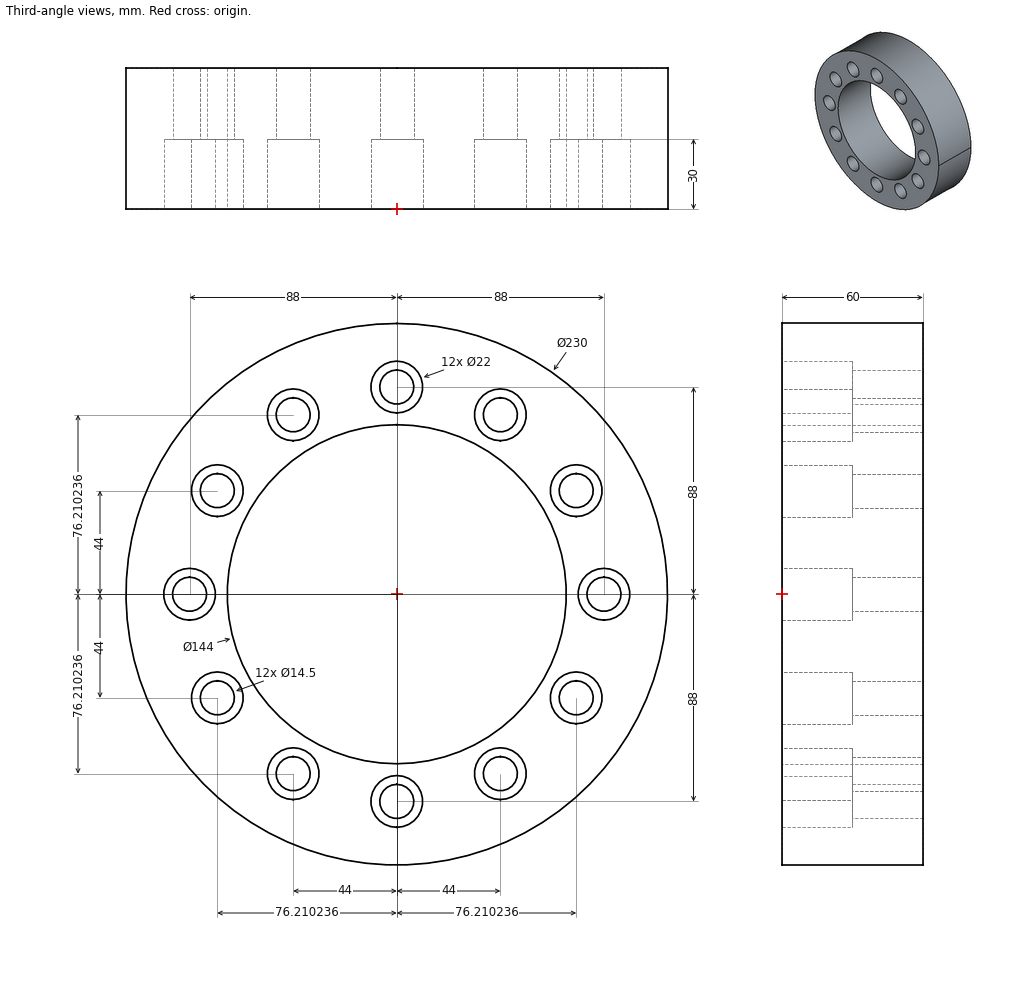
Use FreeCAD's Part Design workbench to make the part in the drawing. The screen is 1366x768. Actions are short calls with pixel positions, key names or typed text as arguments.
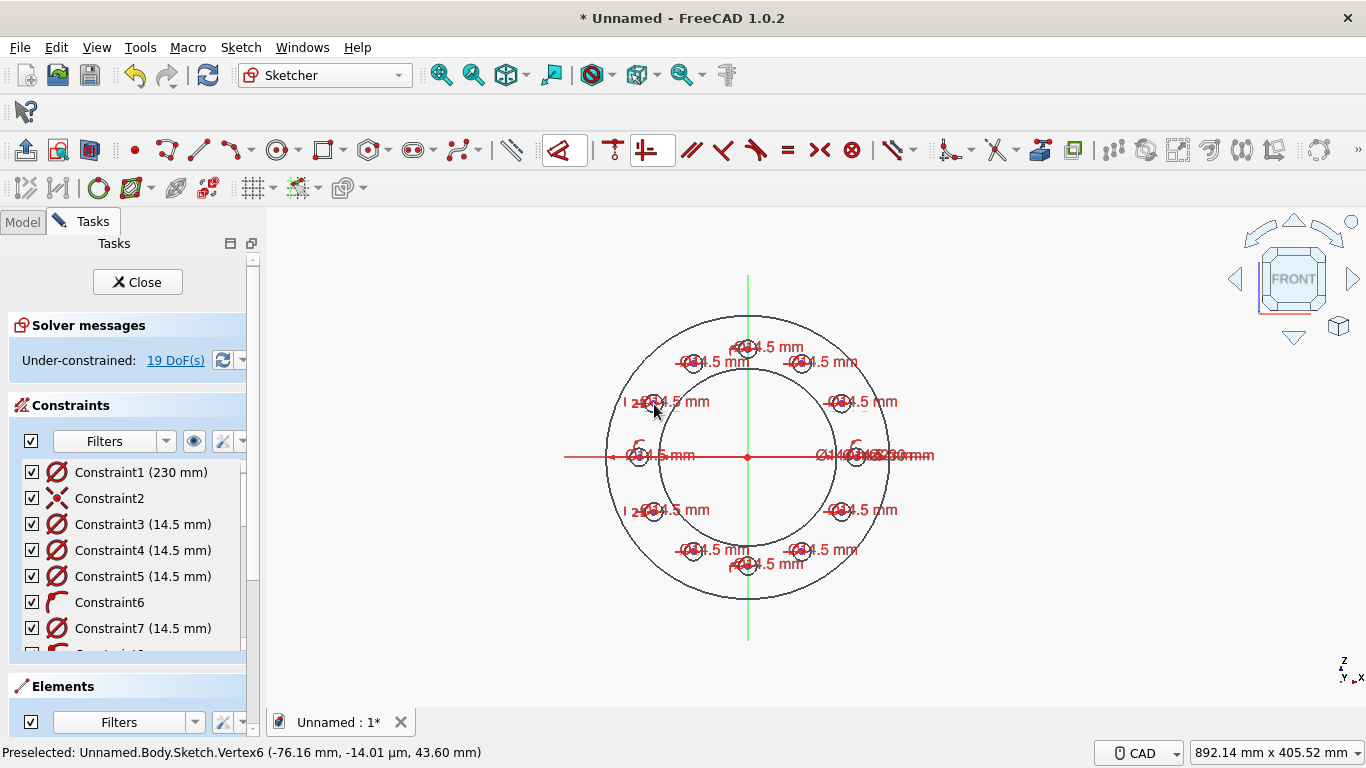
click(694, 552)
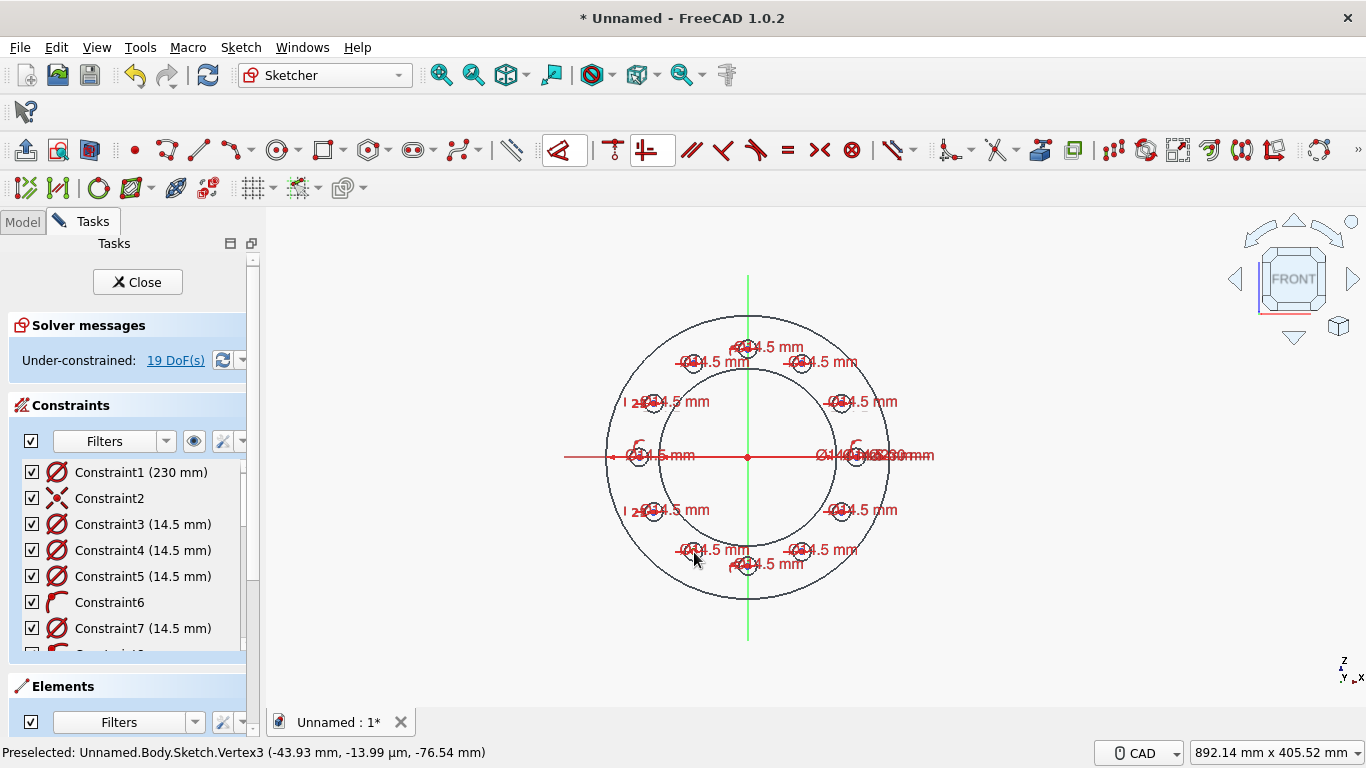
click(694, 364)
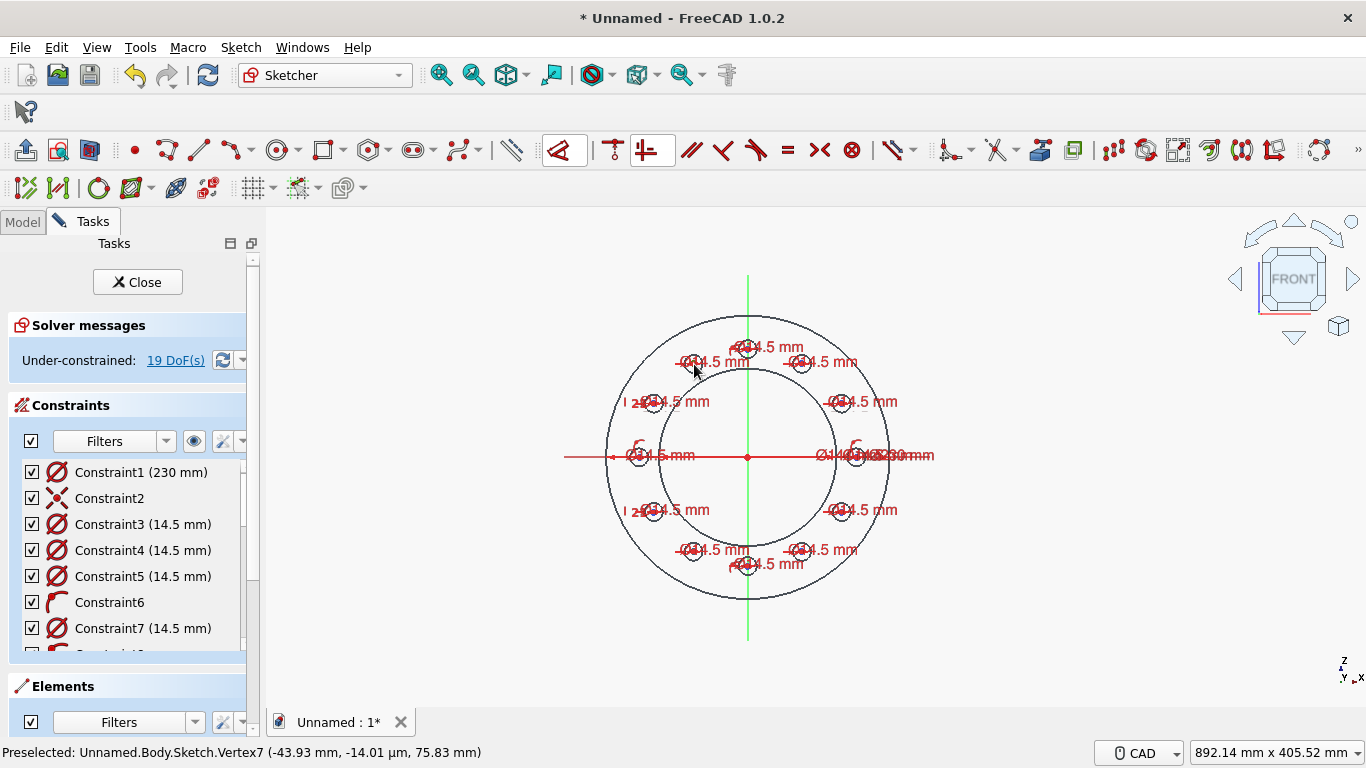
key(v)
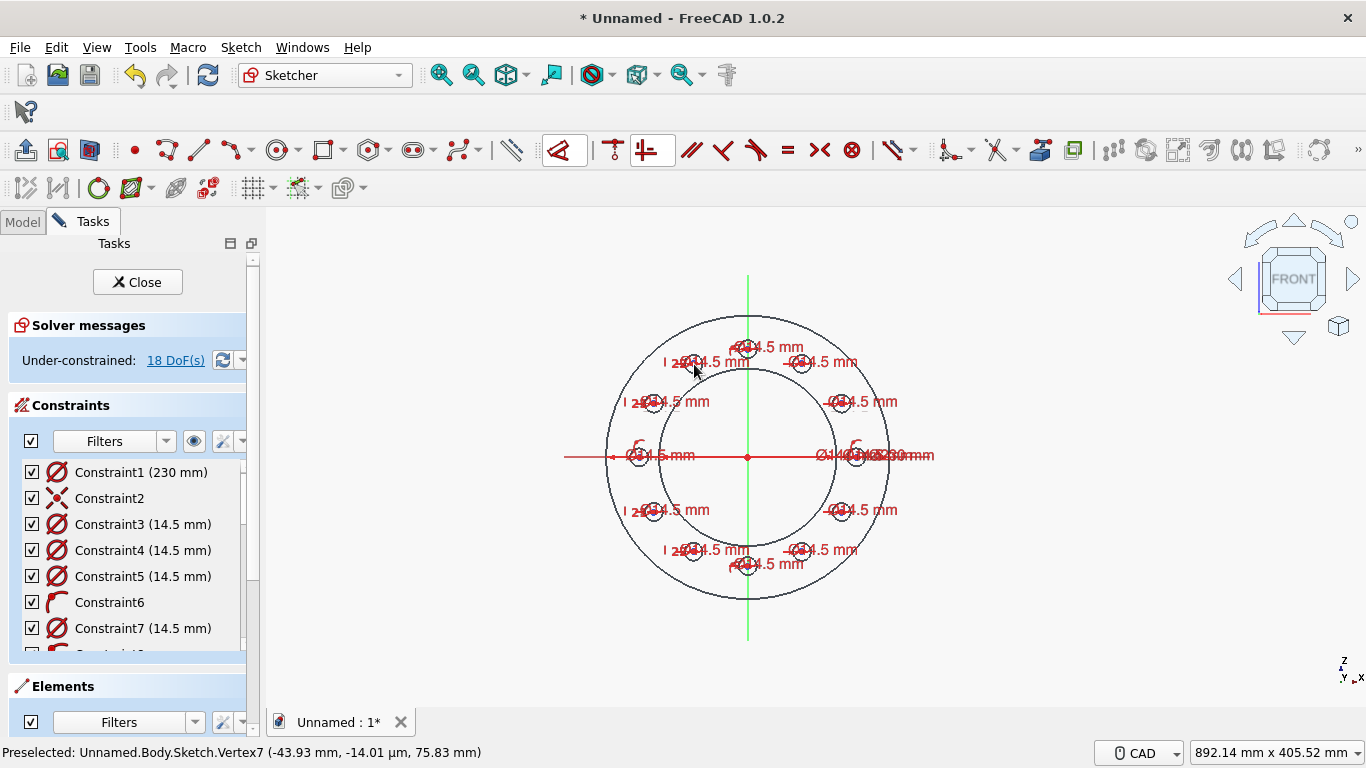
click(694, 552)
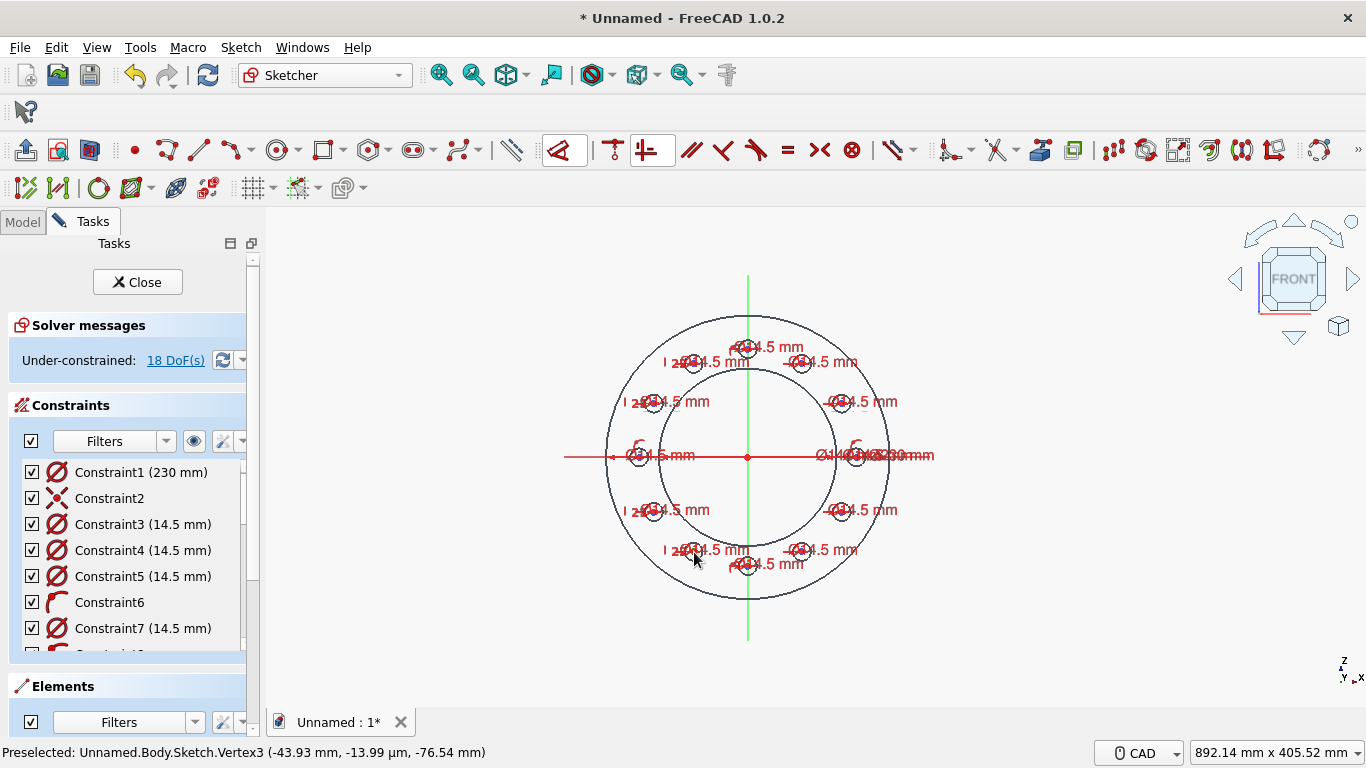
click(802, 552)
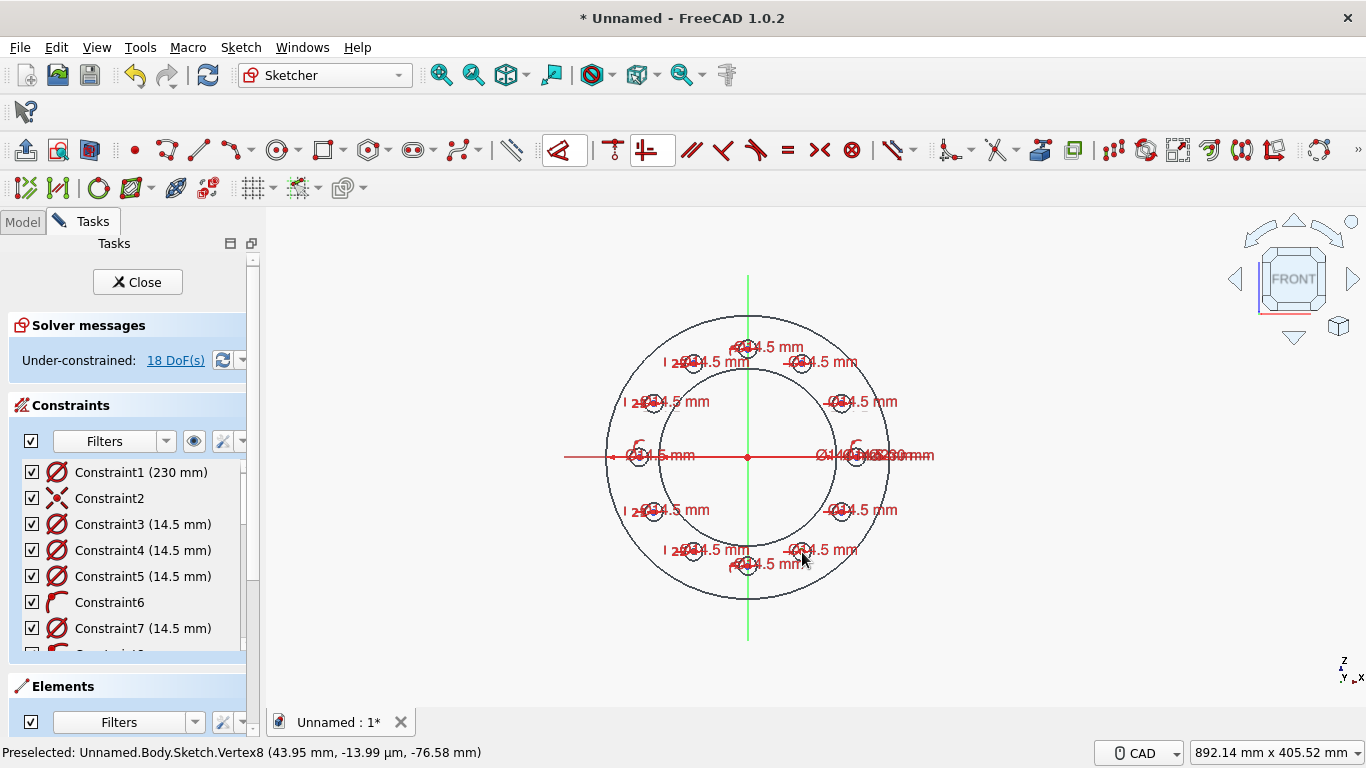
key(h)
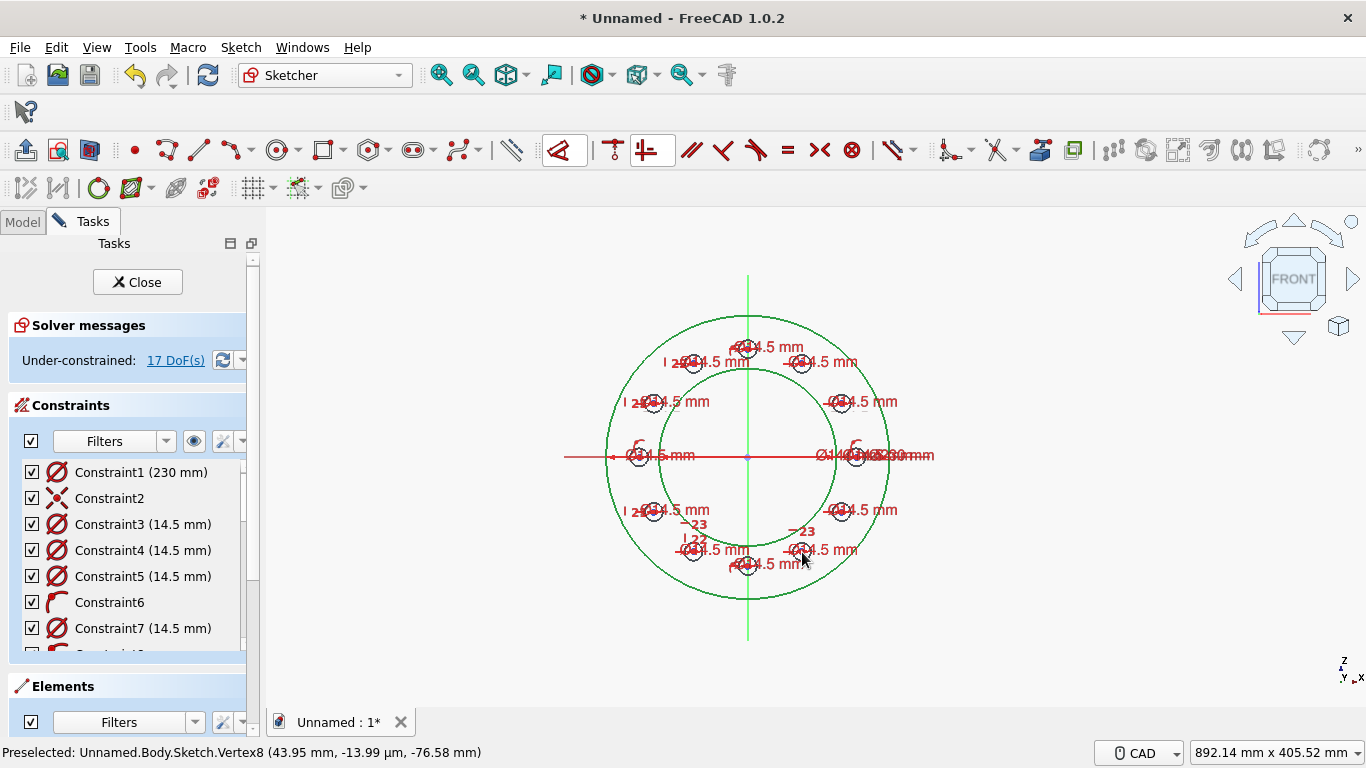
click(654, 512)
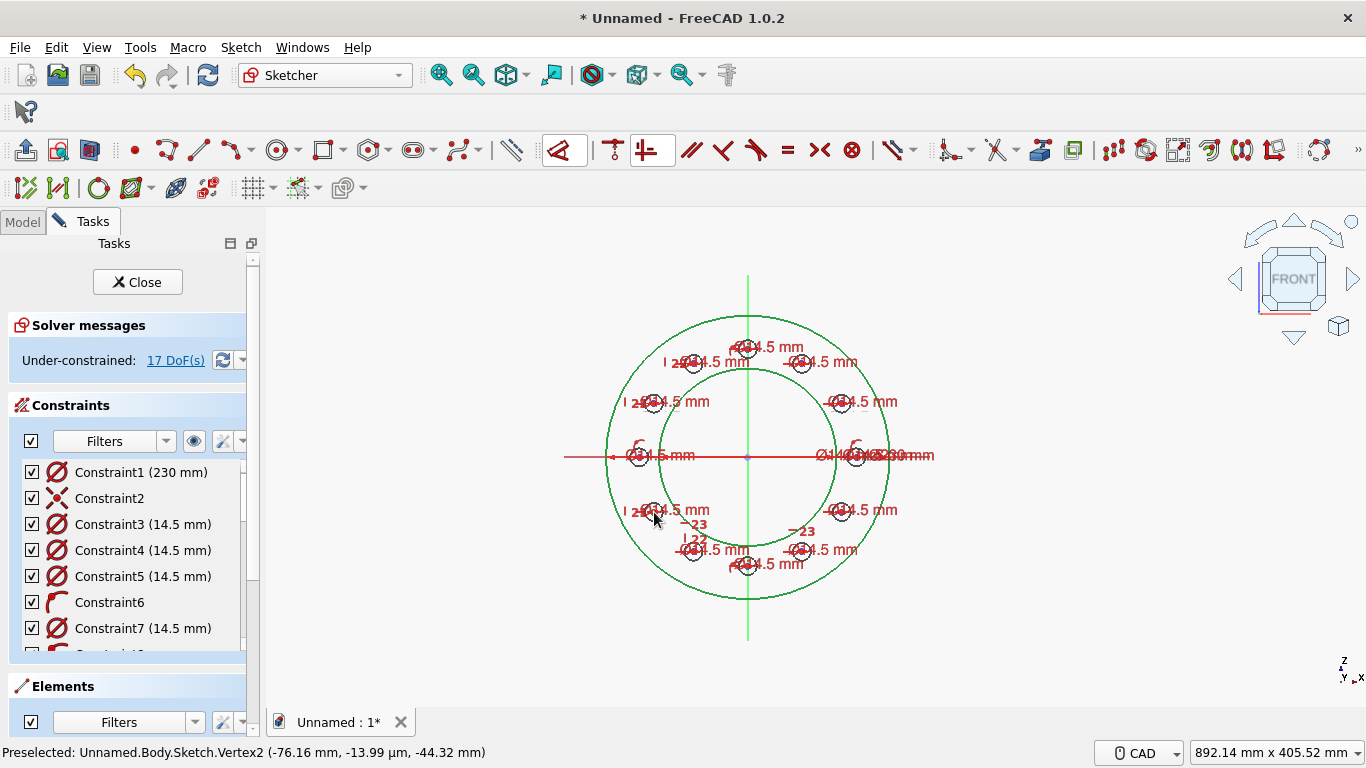
click(842, 512)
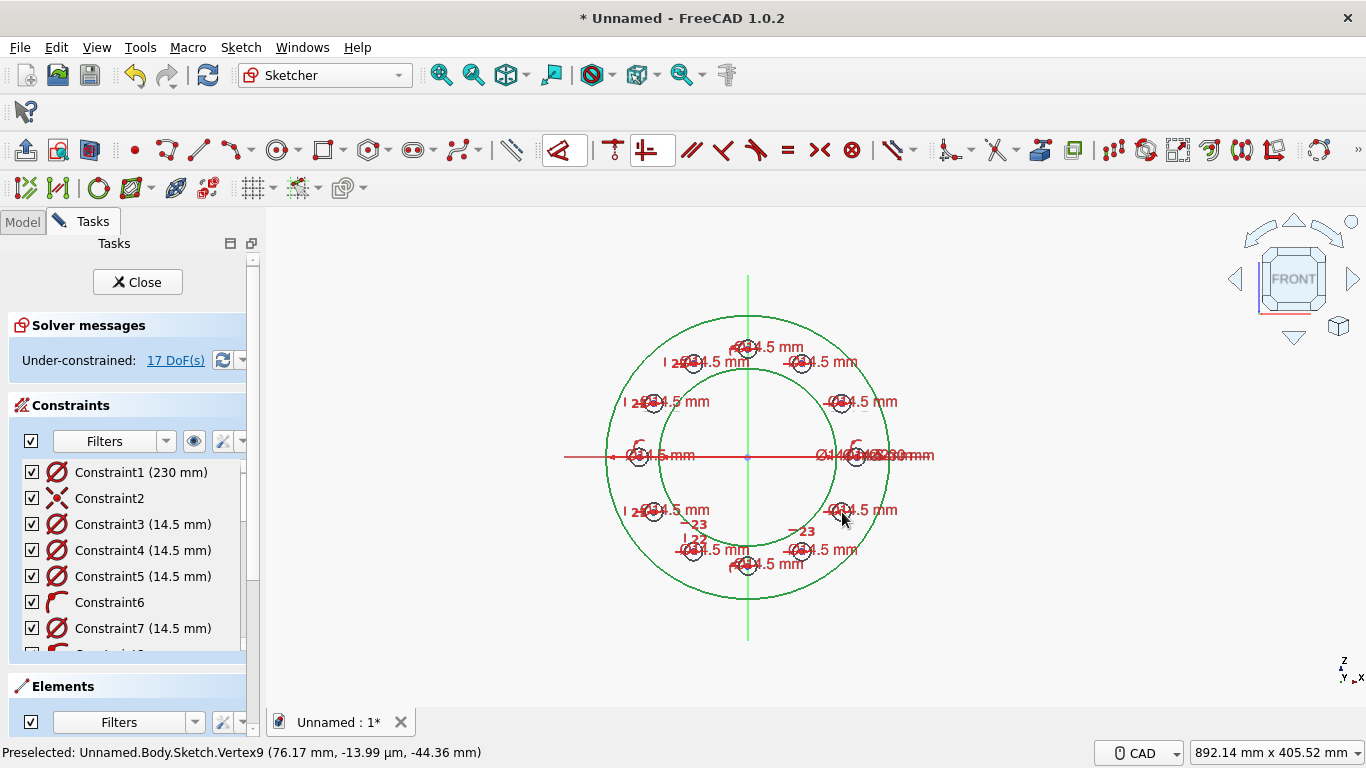
click(670, 150)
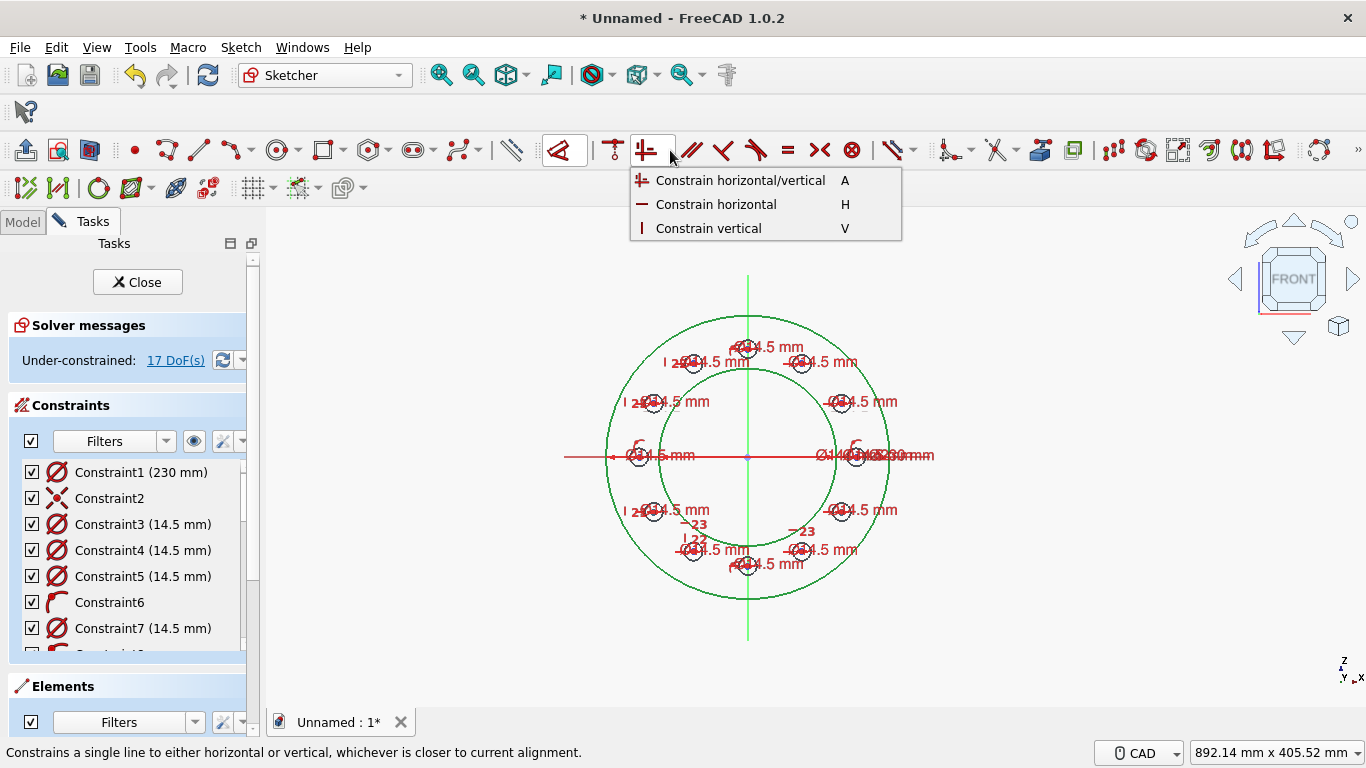
click(766, 204)